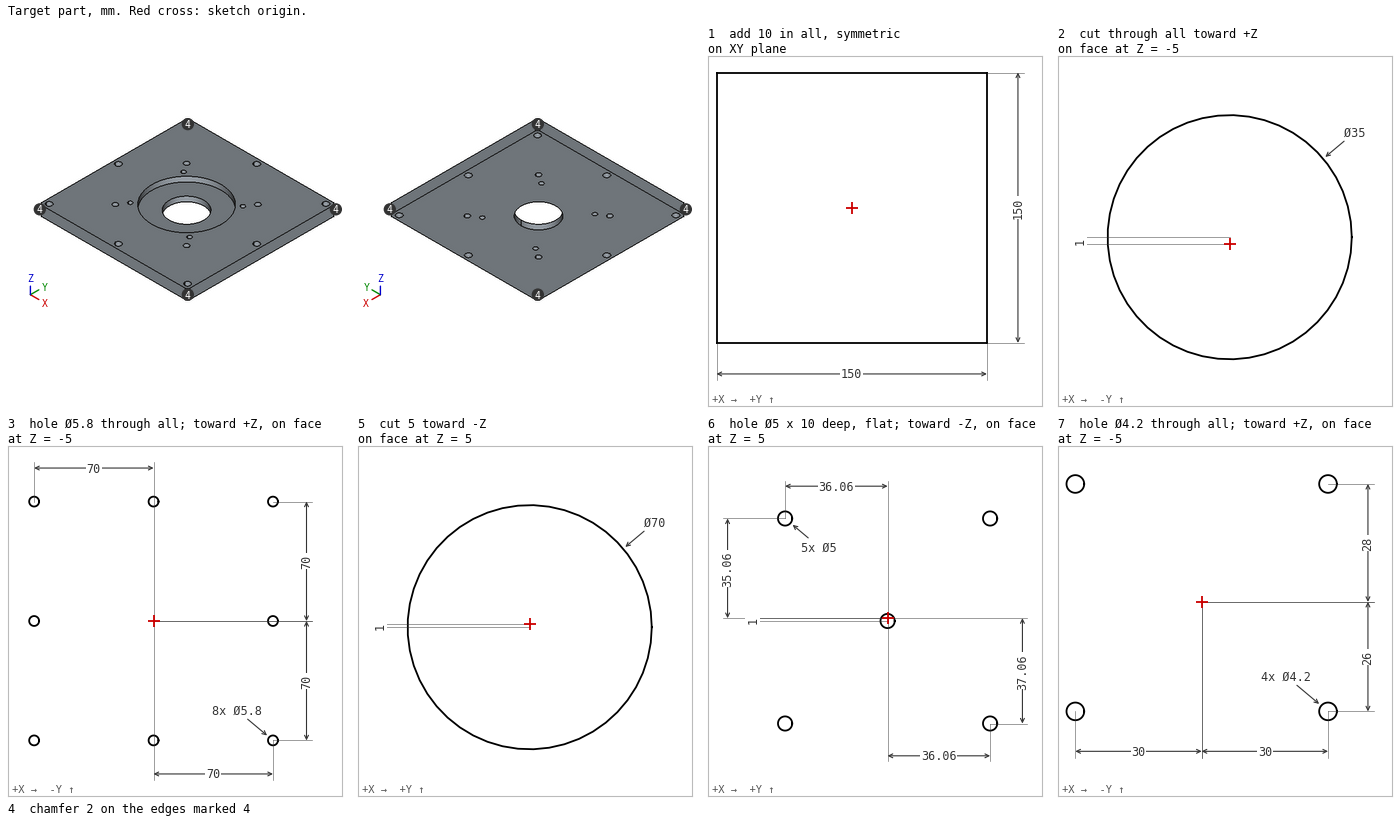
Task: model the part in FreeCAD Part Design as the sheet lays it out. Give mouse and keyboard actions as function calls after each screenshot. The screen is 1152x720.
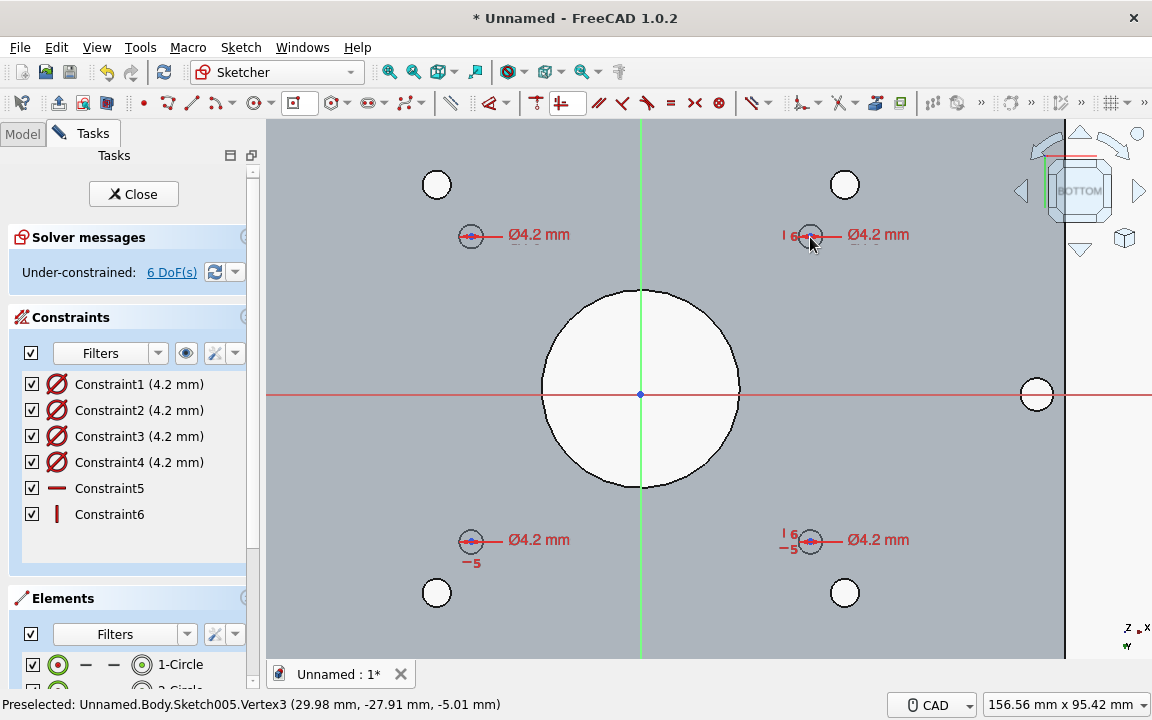
click(471, 542)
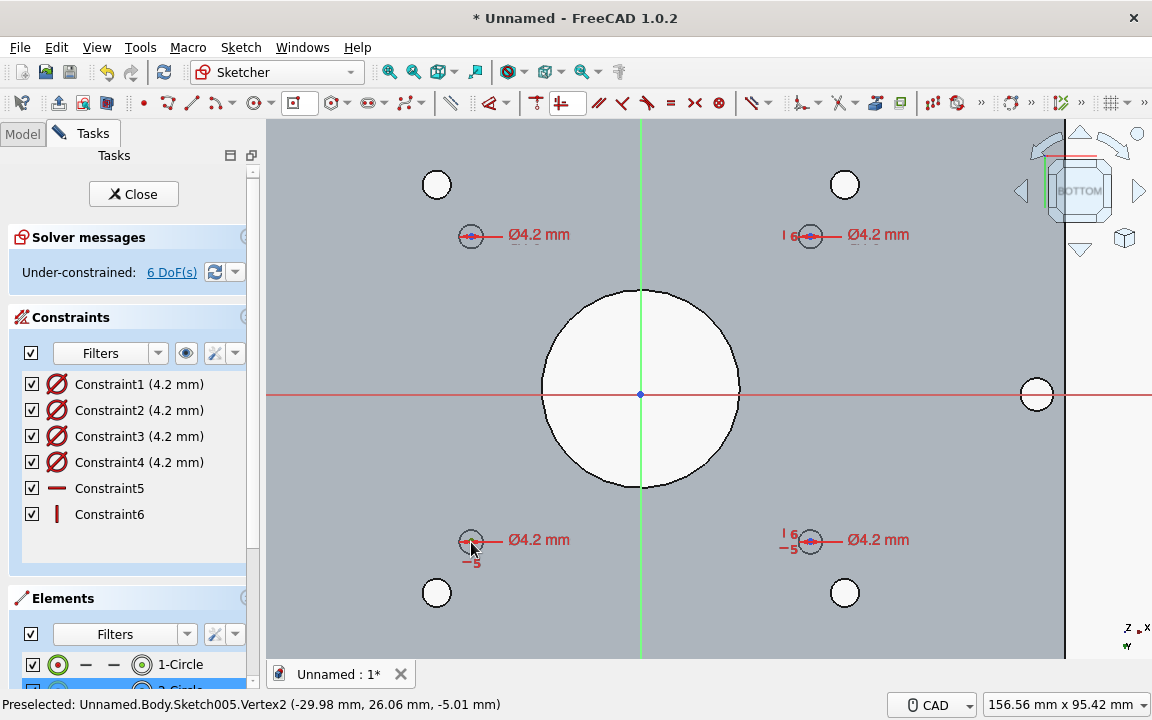
click(471, 237)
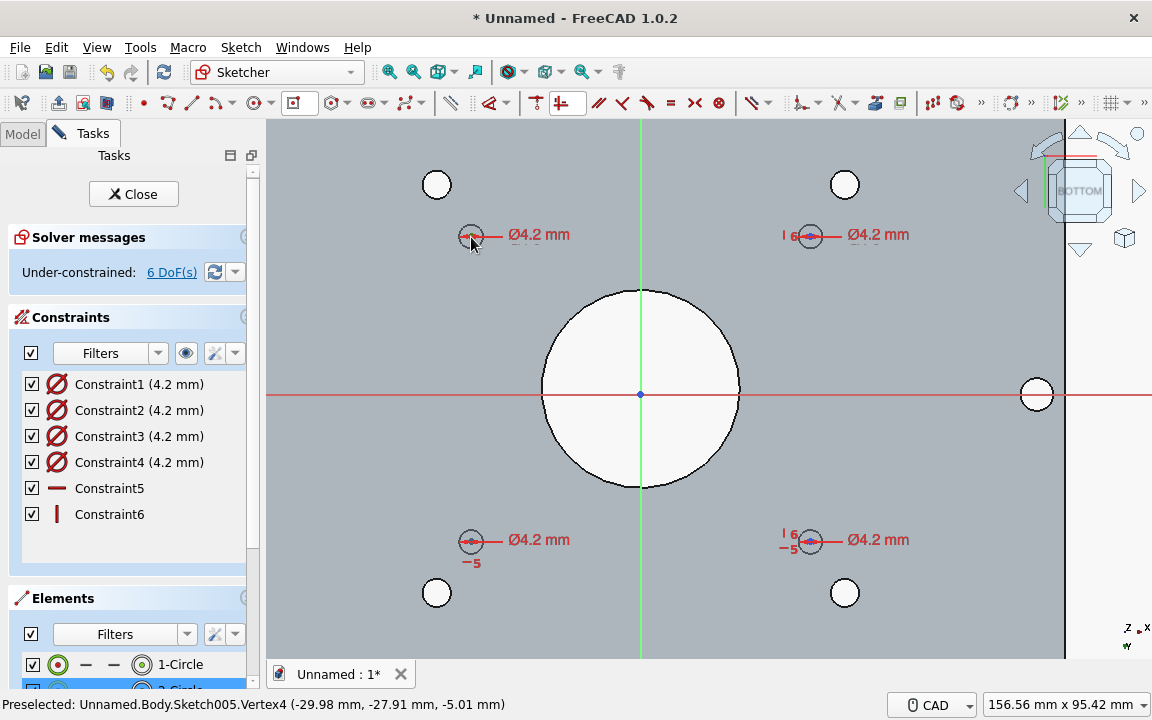
key(v)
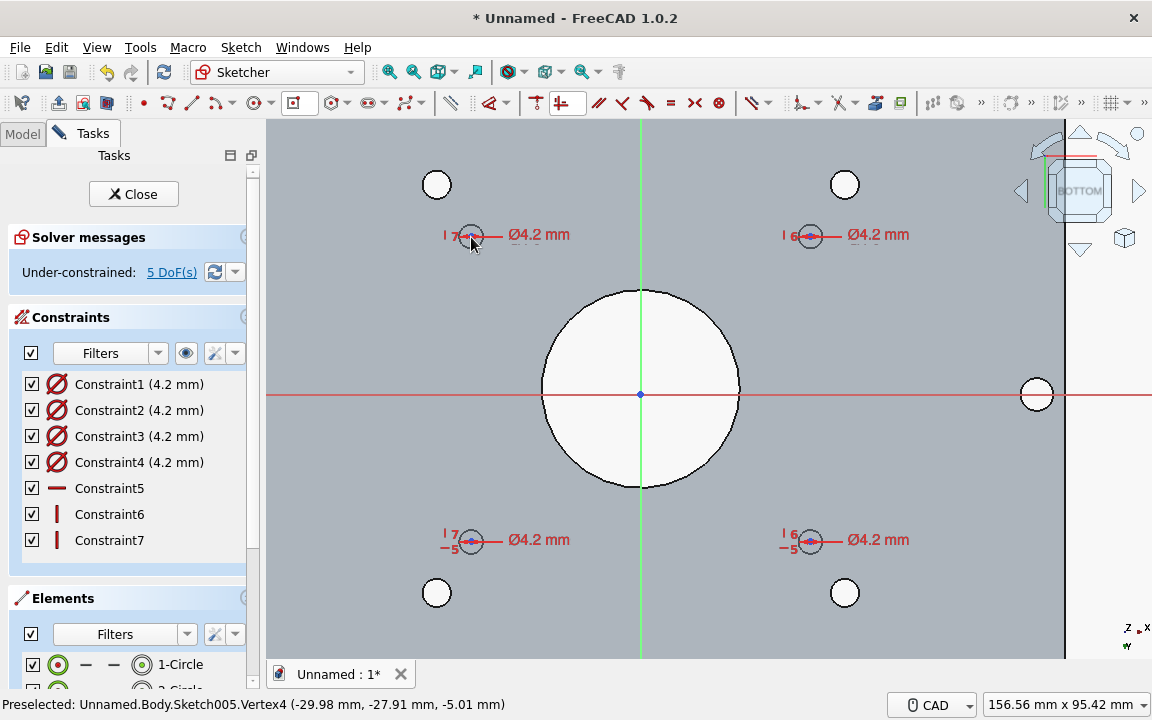
click(810, 237)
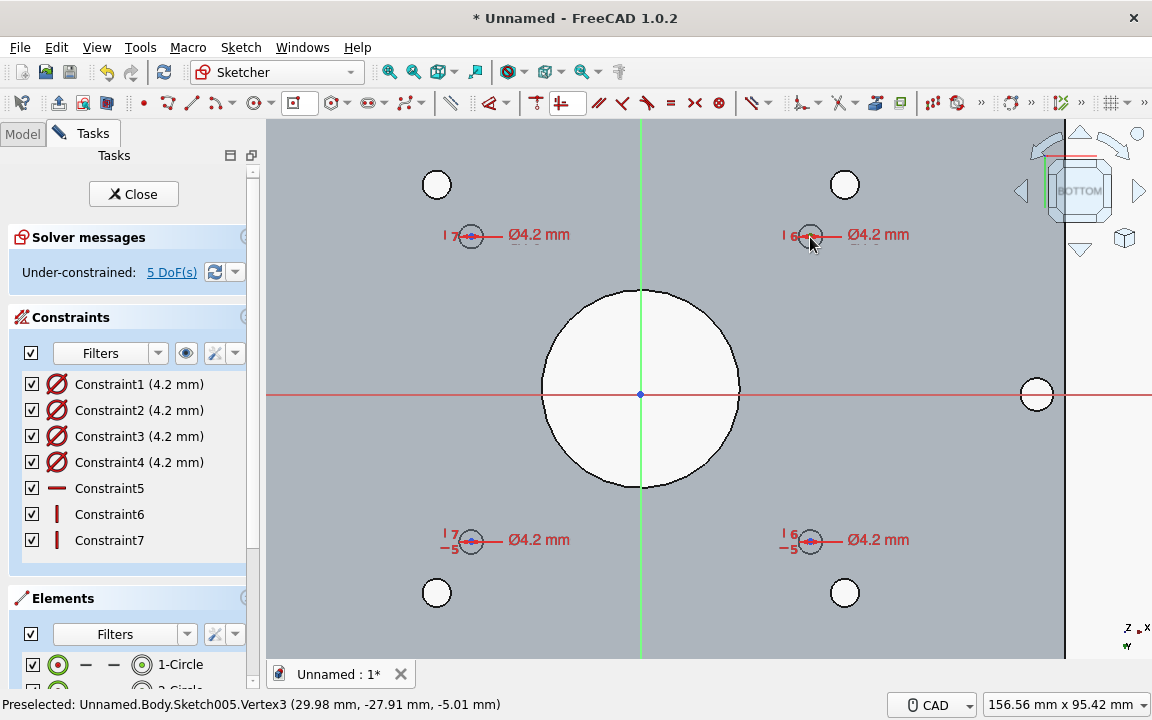
click(471, 237)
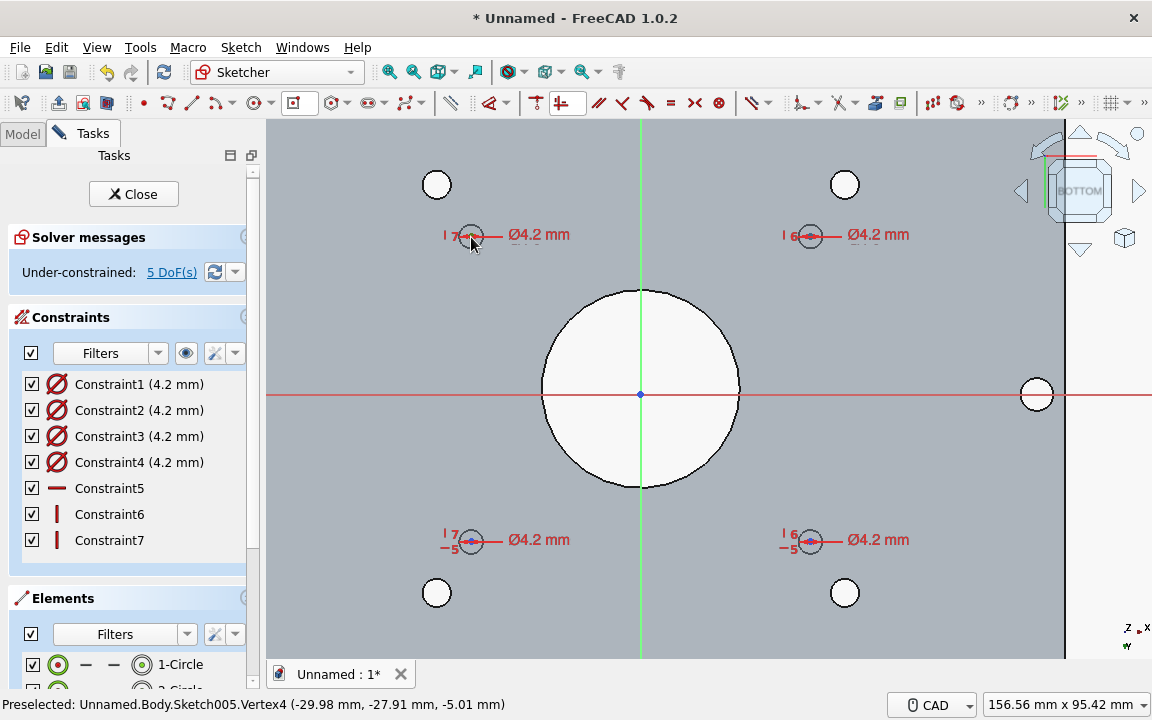
key(h)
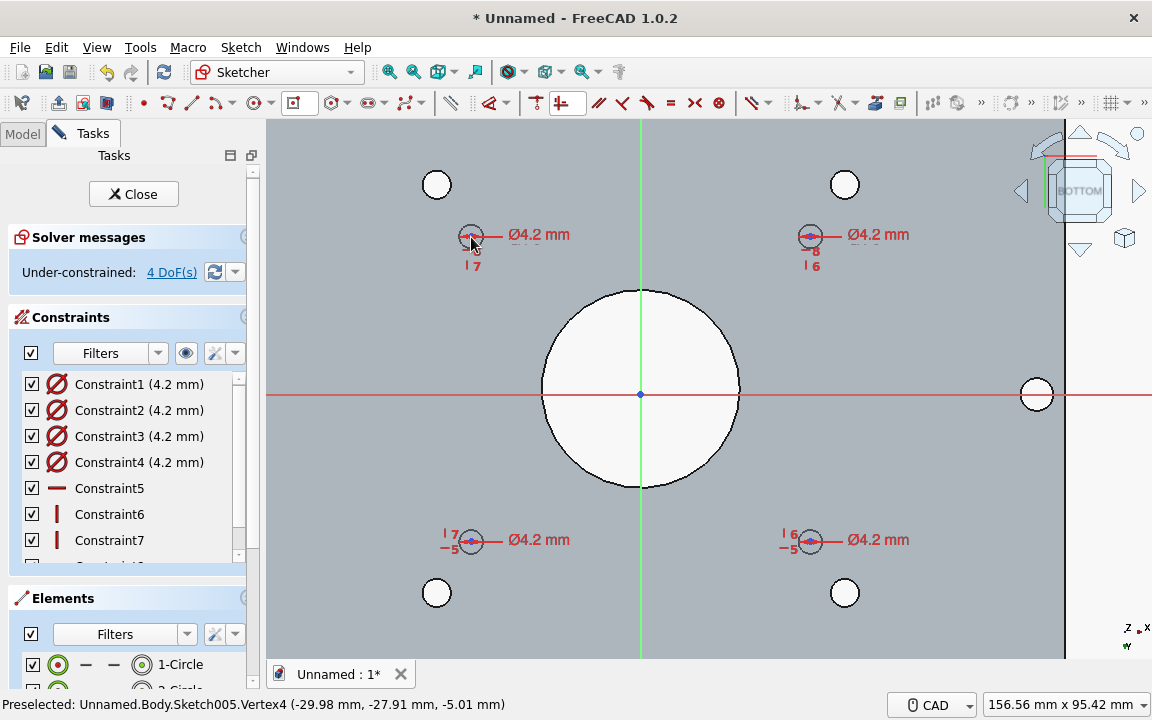
click(490, 104)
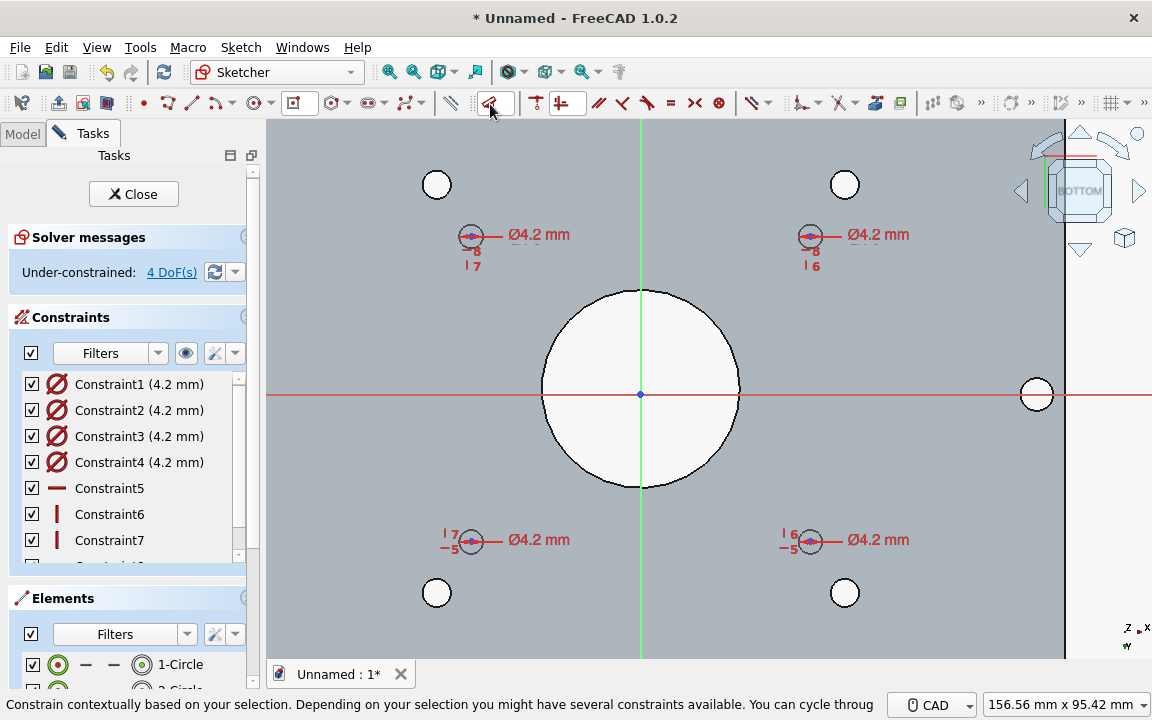
click(810, 542)
click(726, 576)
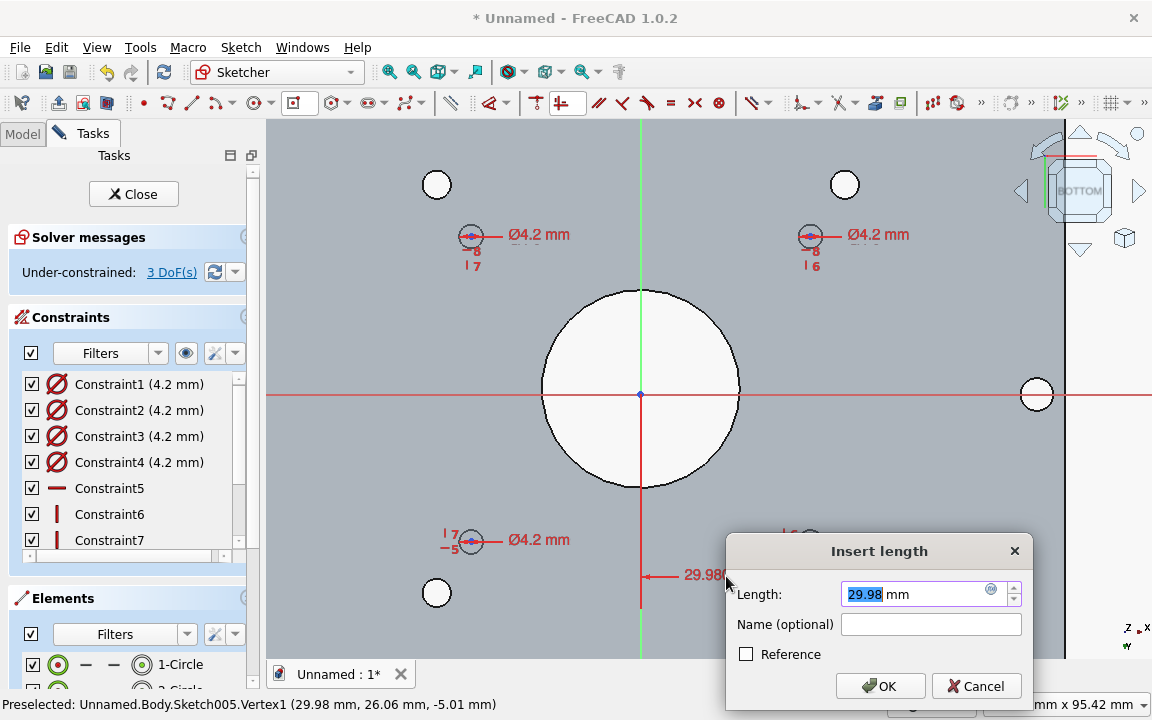
text(30)
key(Return)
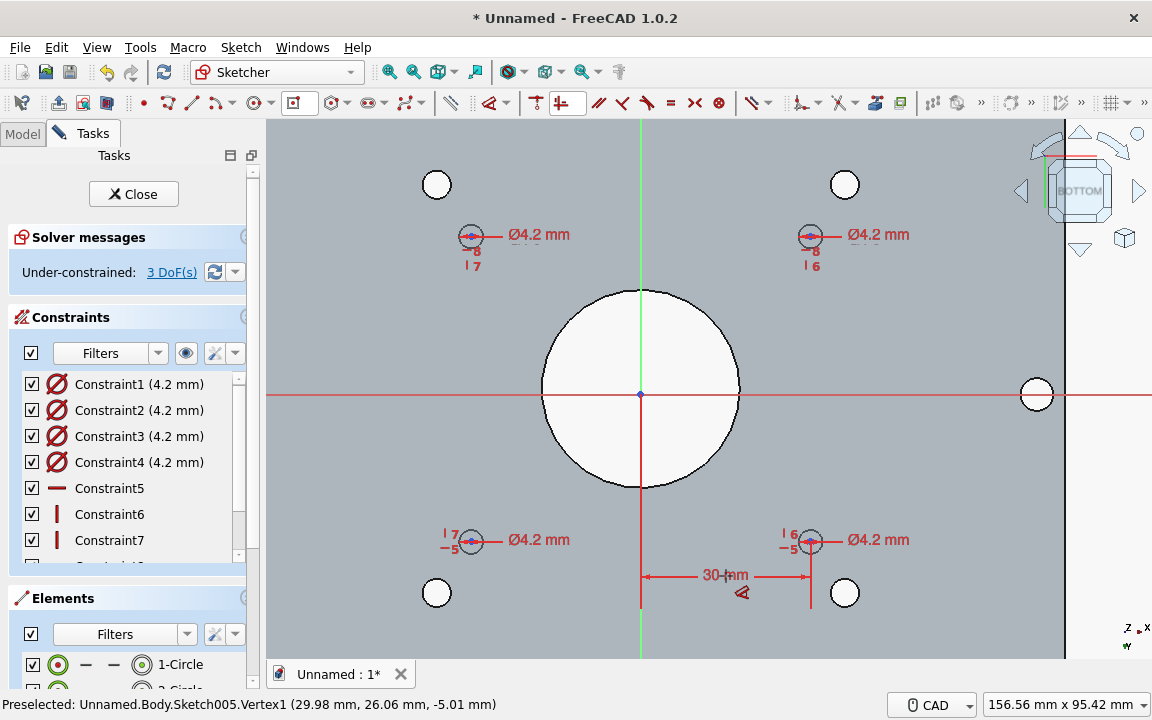
click(811, 542)
click(845, 468)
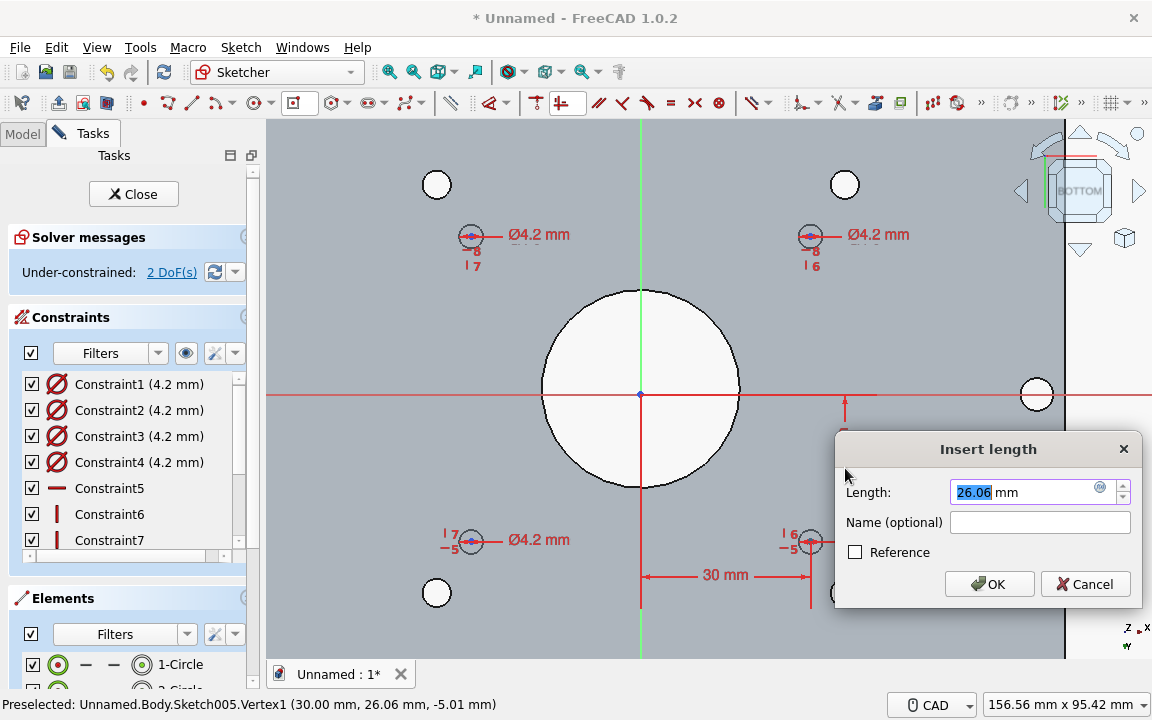
text(26)
key(Return)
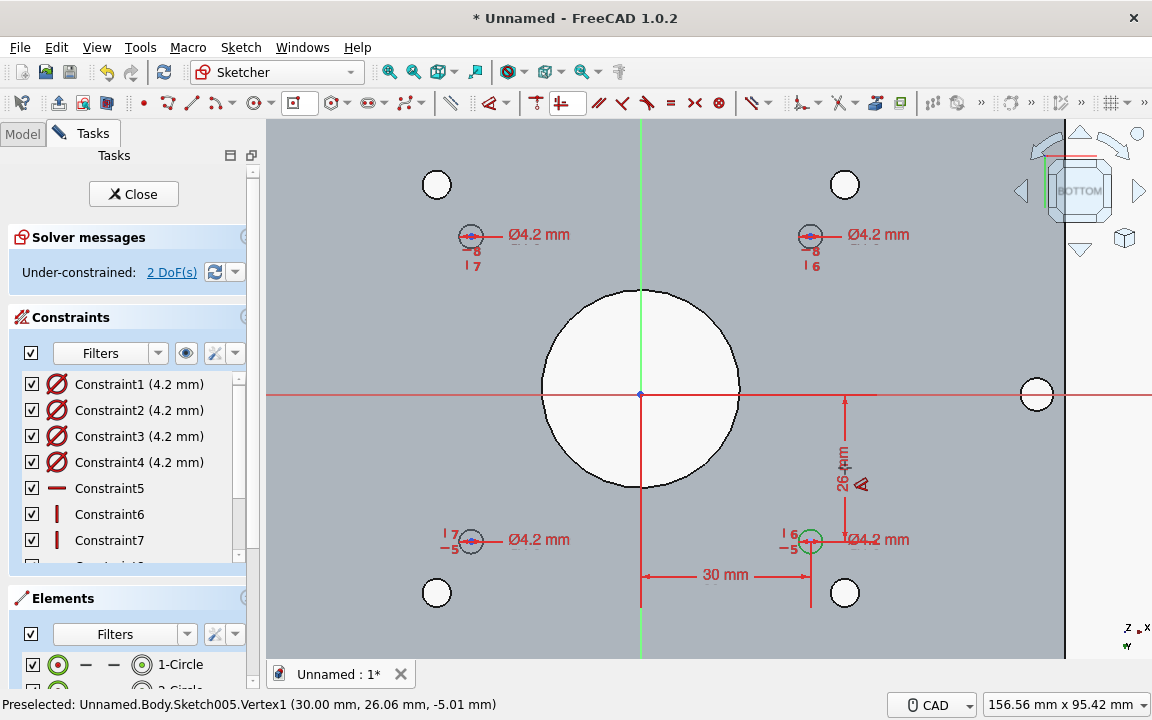
click(471, 542)
click(556, 576)